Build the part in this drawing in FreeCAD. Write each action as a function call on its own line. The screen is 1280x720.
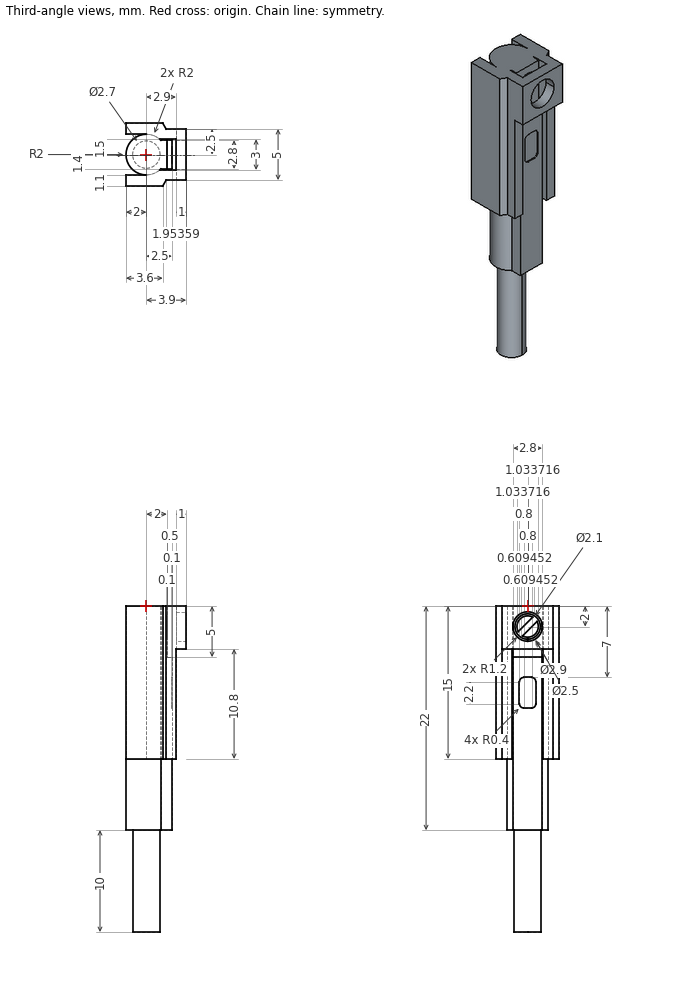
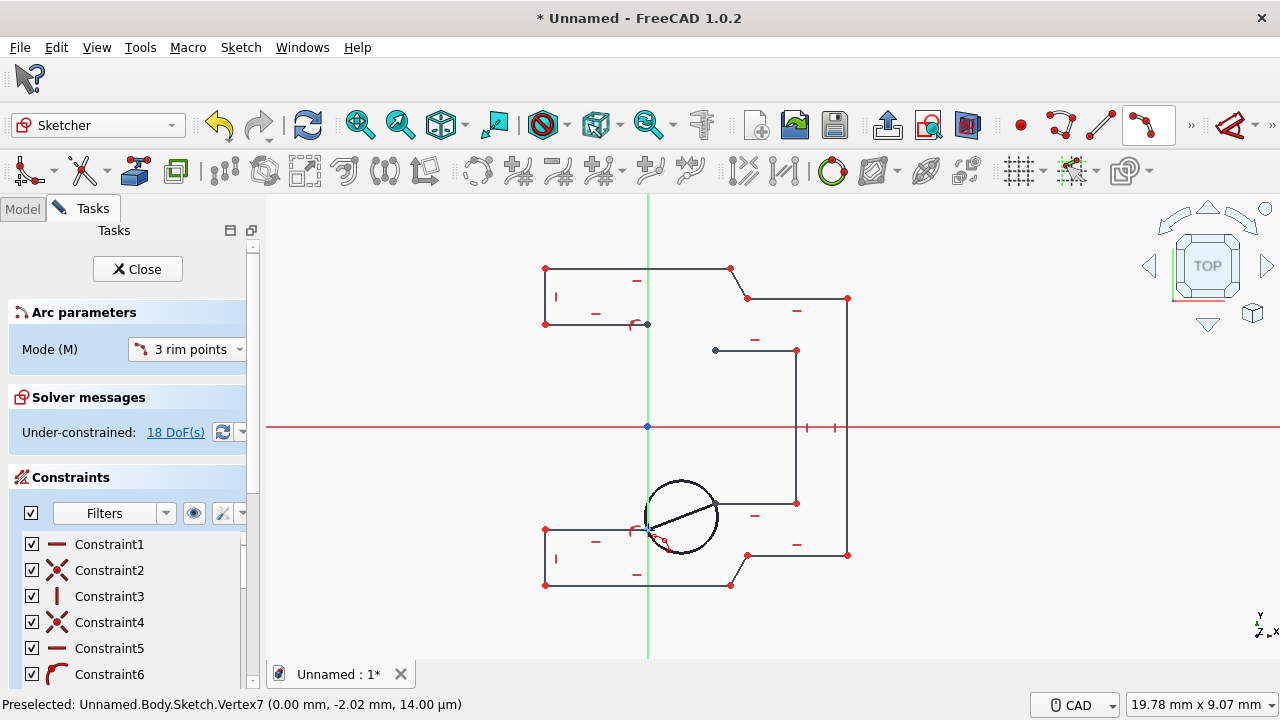
scroll(684, 522, up, 5)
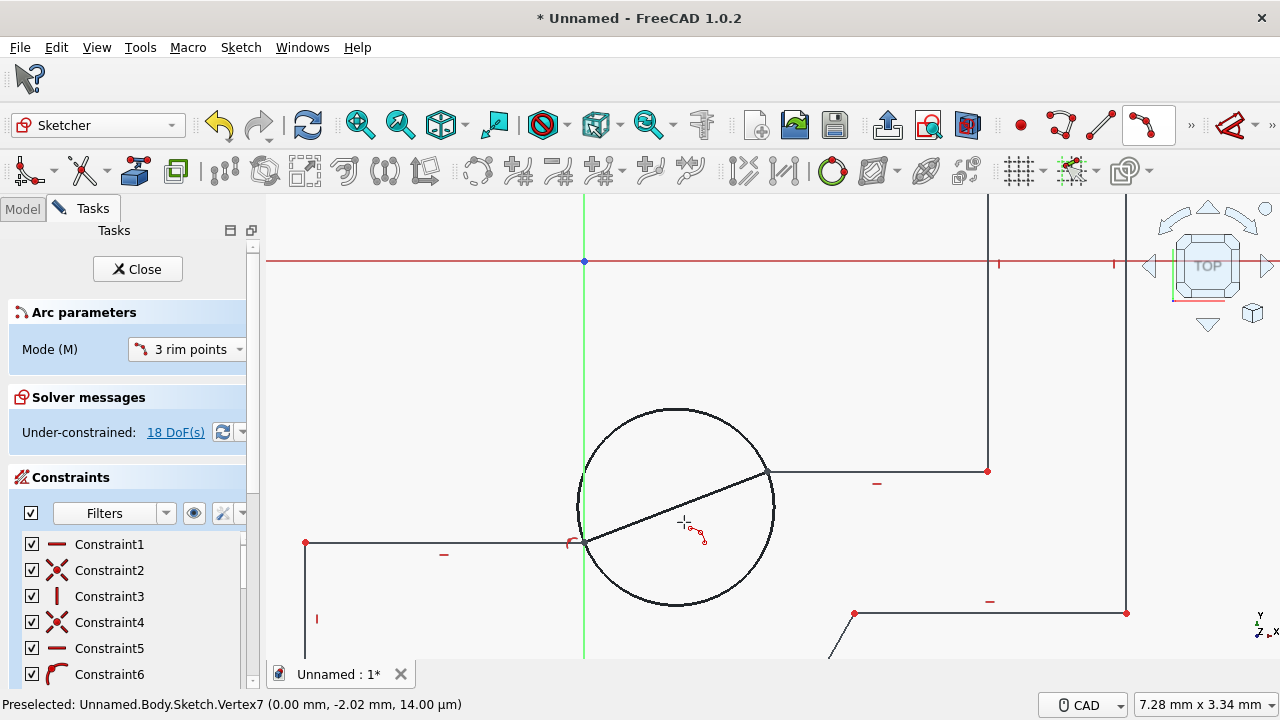
click(683, 522)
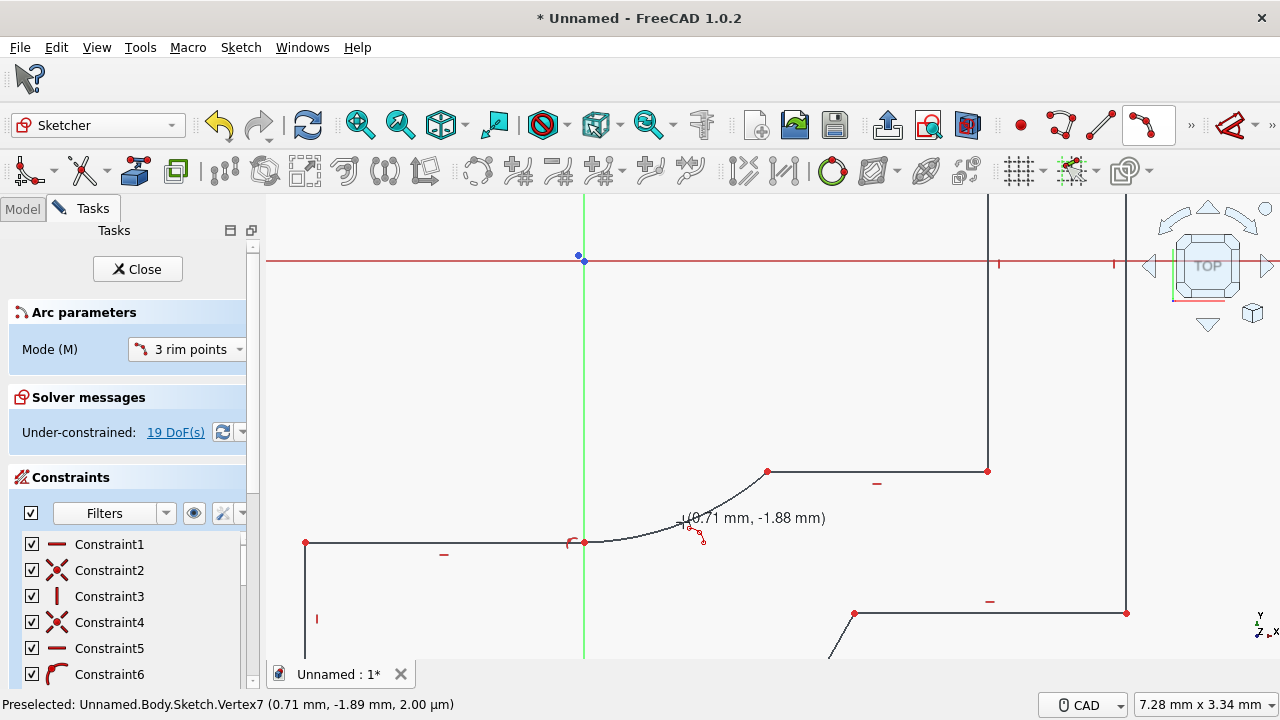
scroll(697, 523, down, 5)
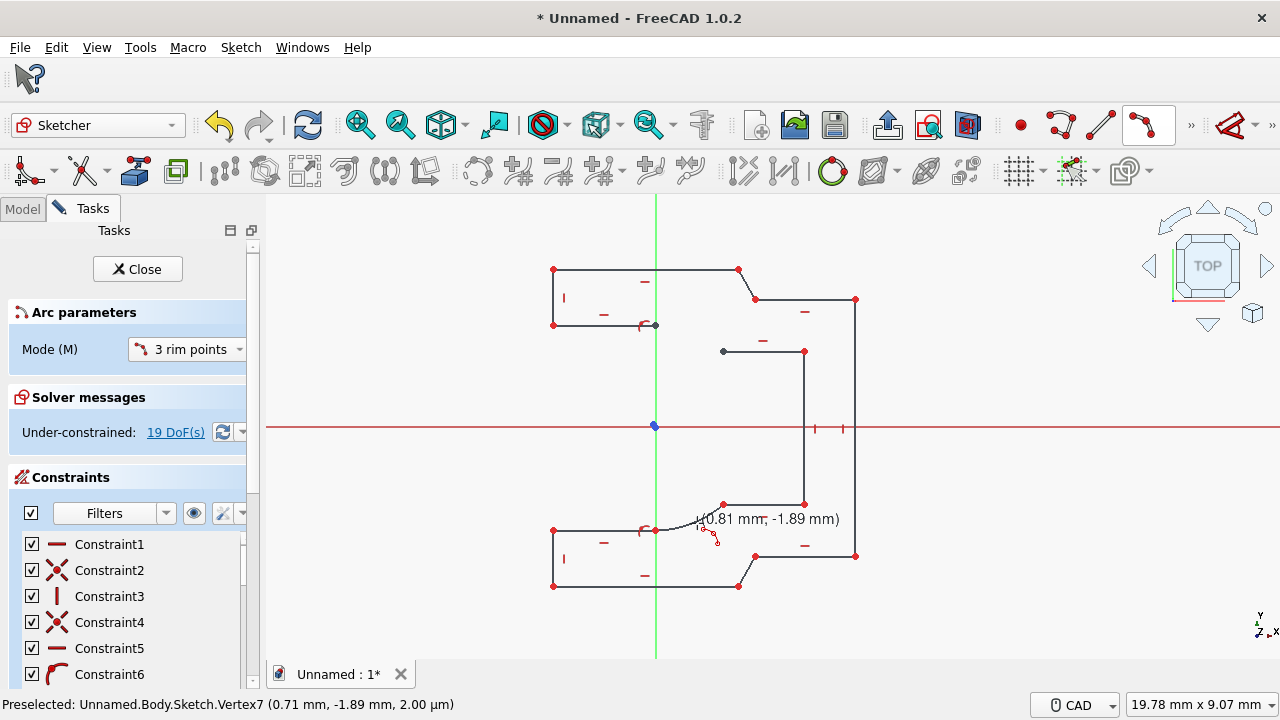
click(656, 326)
click(723, 352)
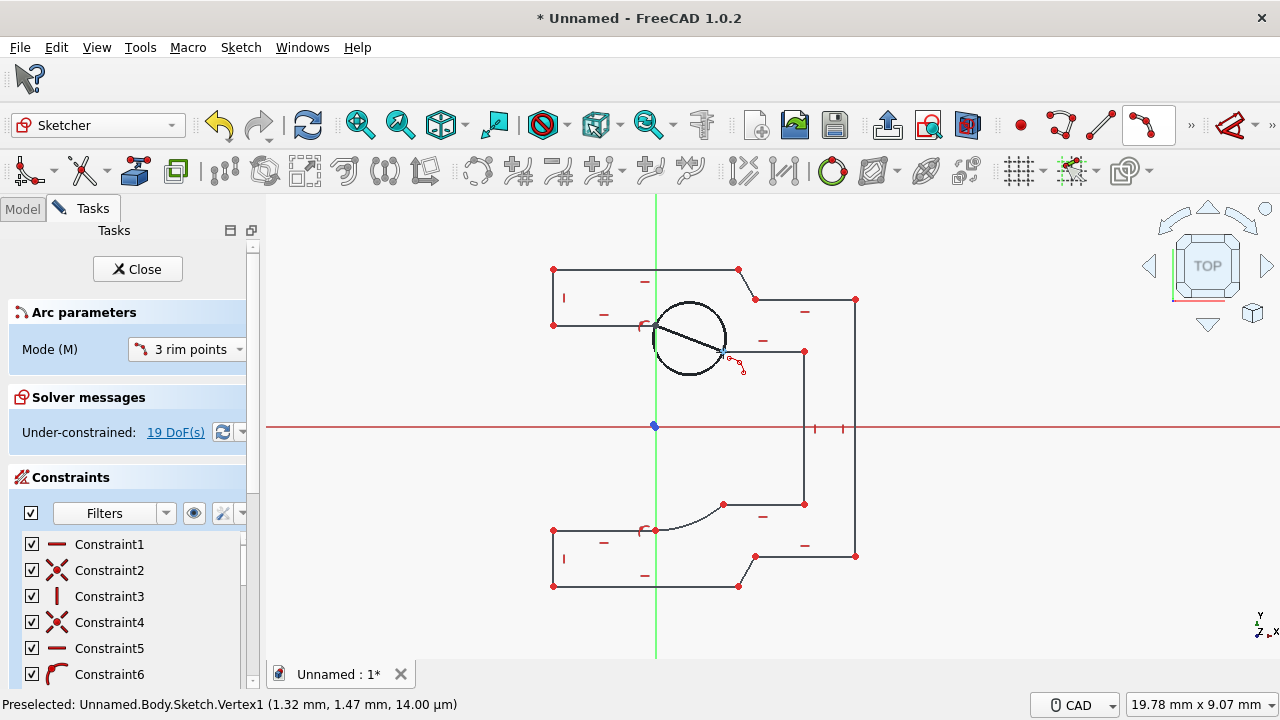
scroll(692, 331, up, 5)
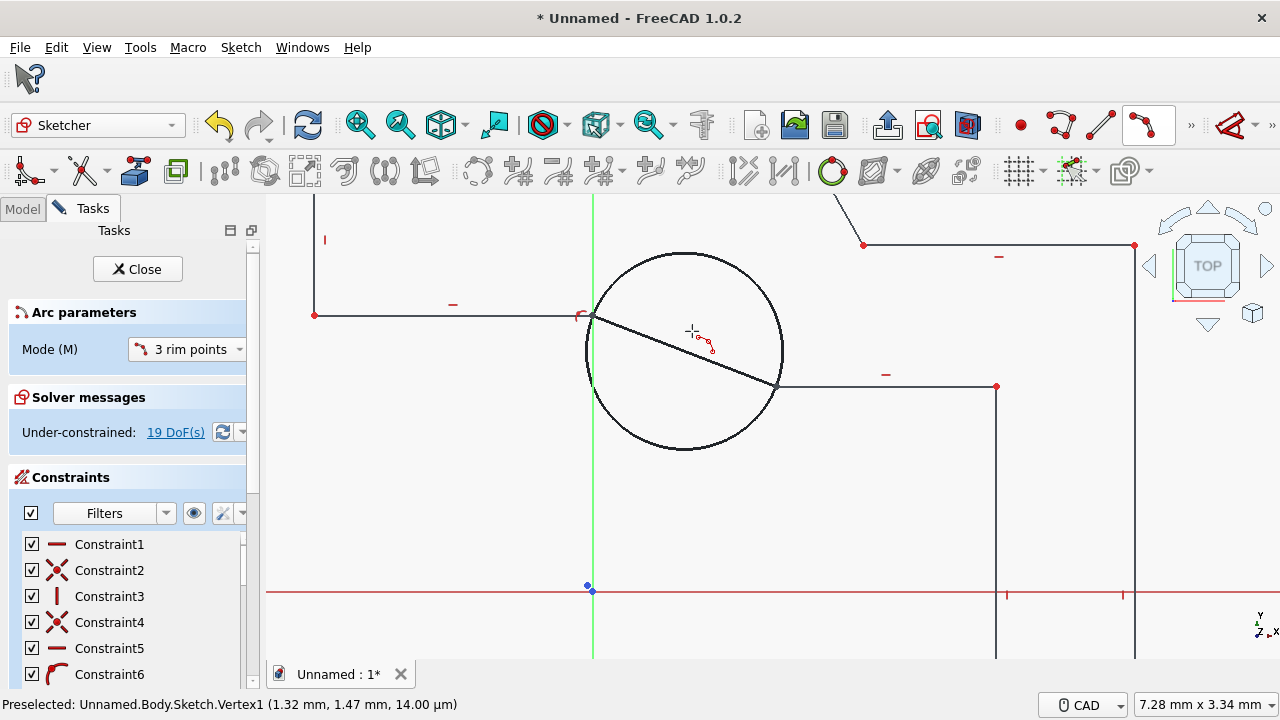
click(691, 331)
key(Escape)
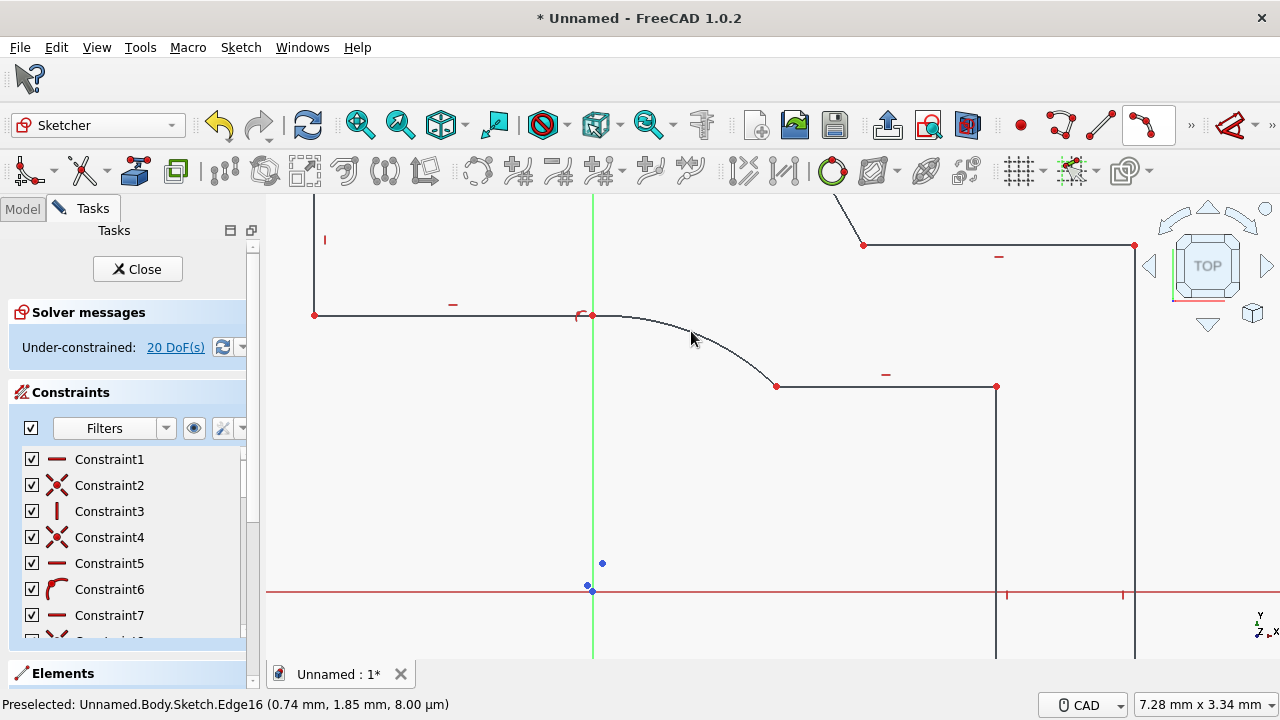
scroll(692, 330, down, 5)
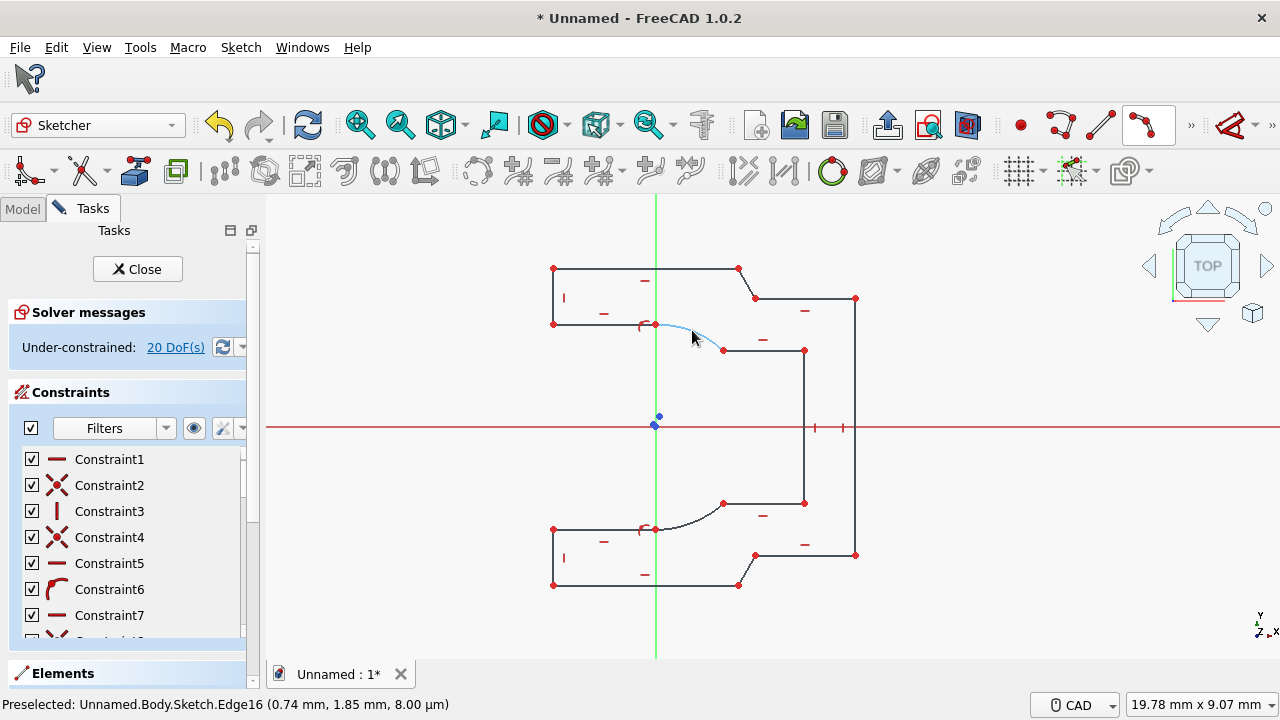
click(625, 530)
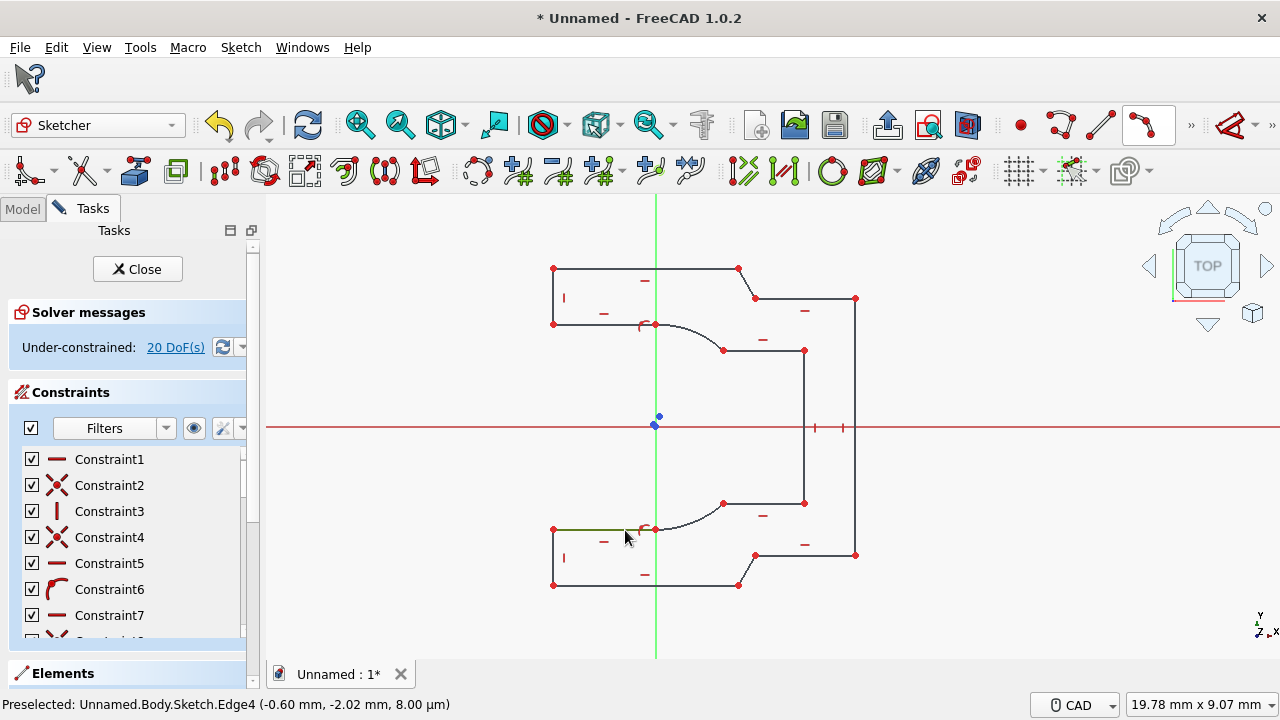
click(678, 527)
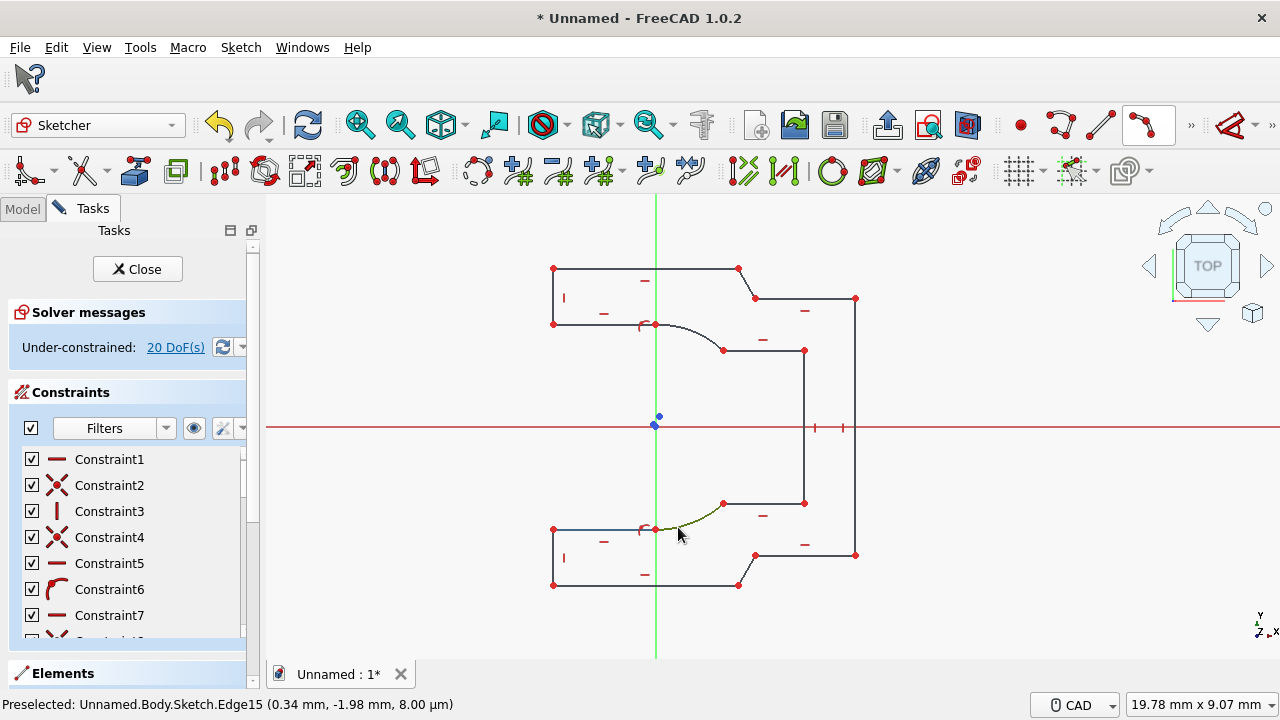
key(t)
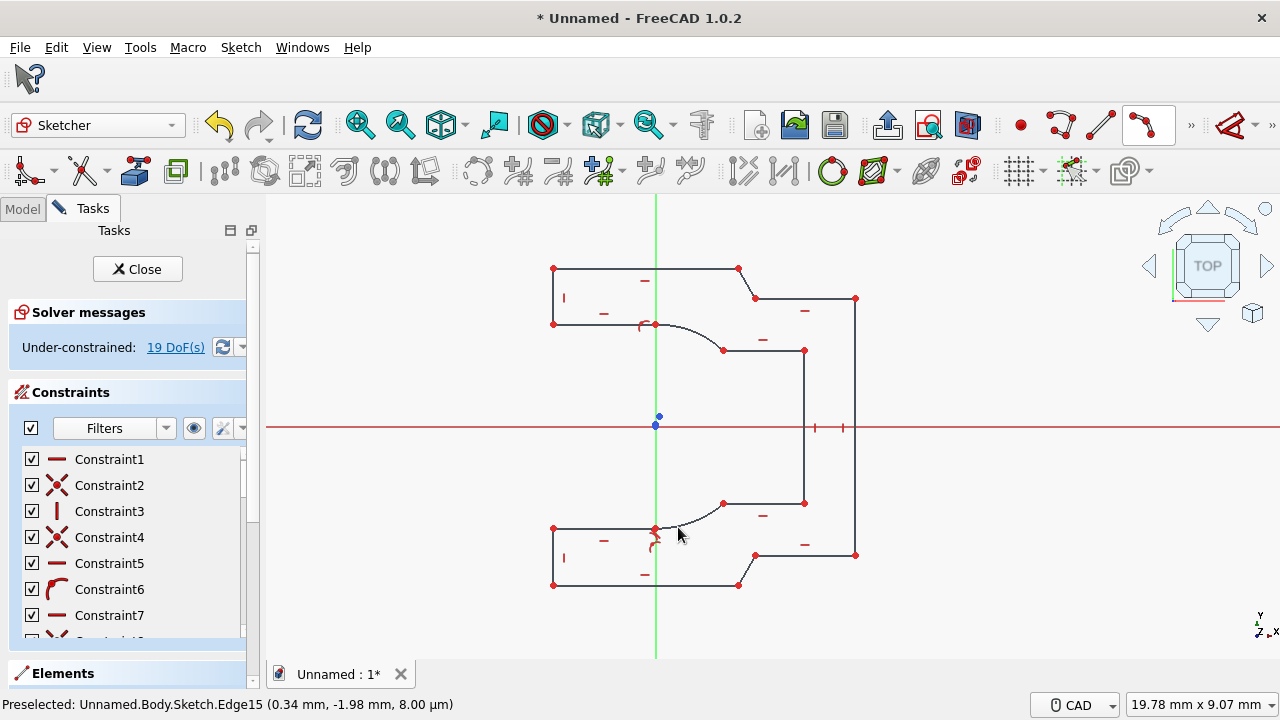
click(584, 325)